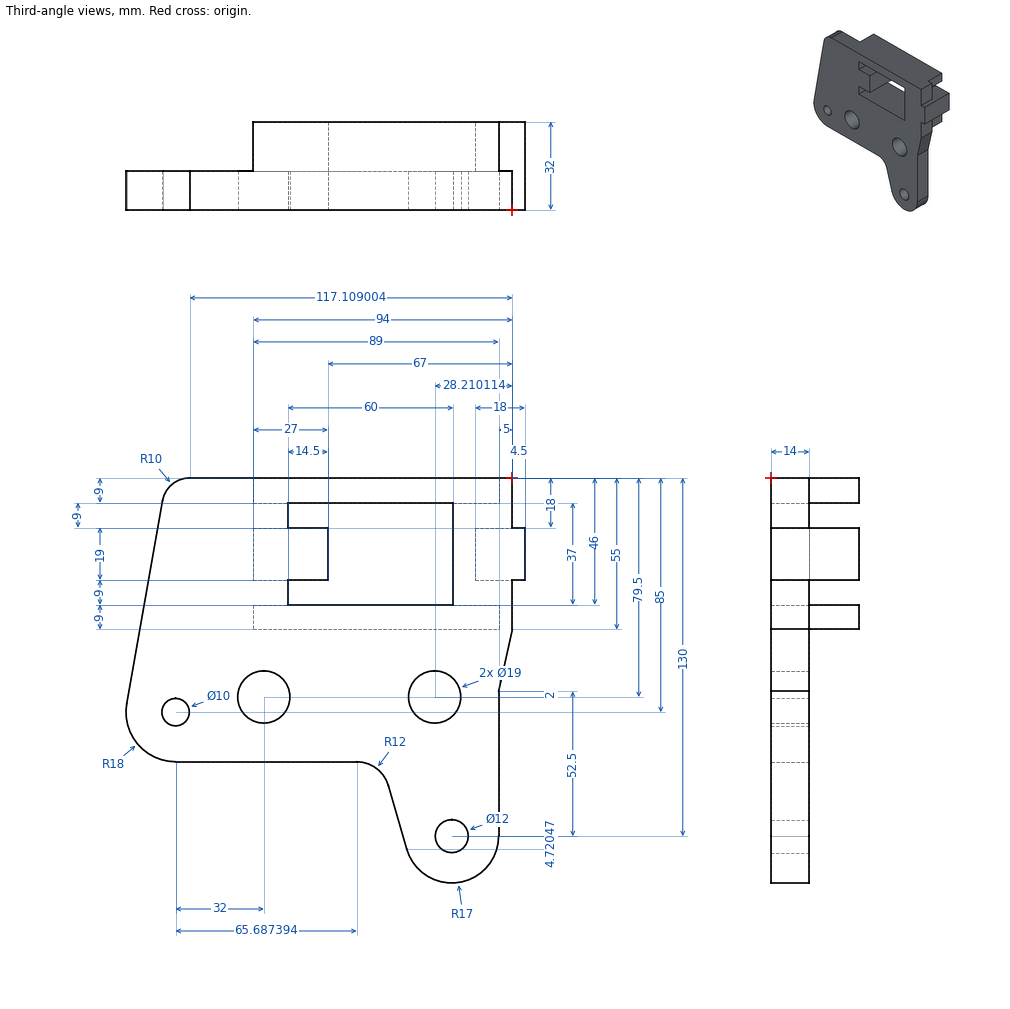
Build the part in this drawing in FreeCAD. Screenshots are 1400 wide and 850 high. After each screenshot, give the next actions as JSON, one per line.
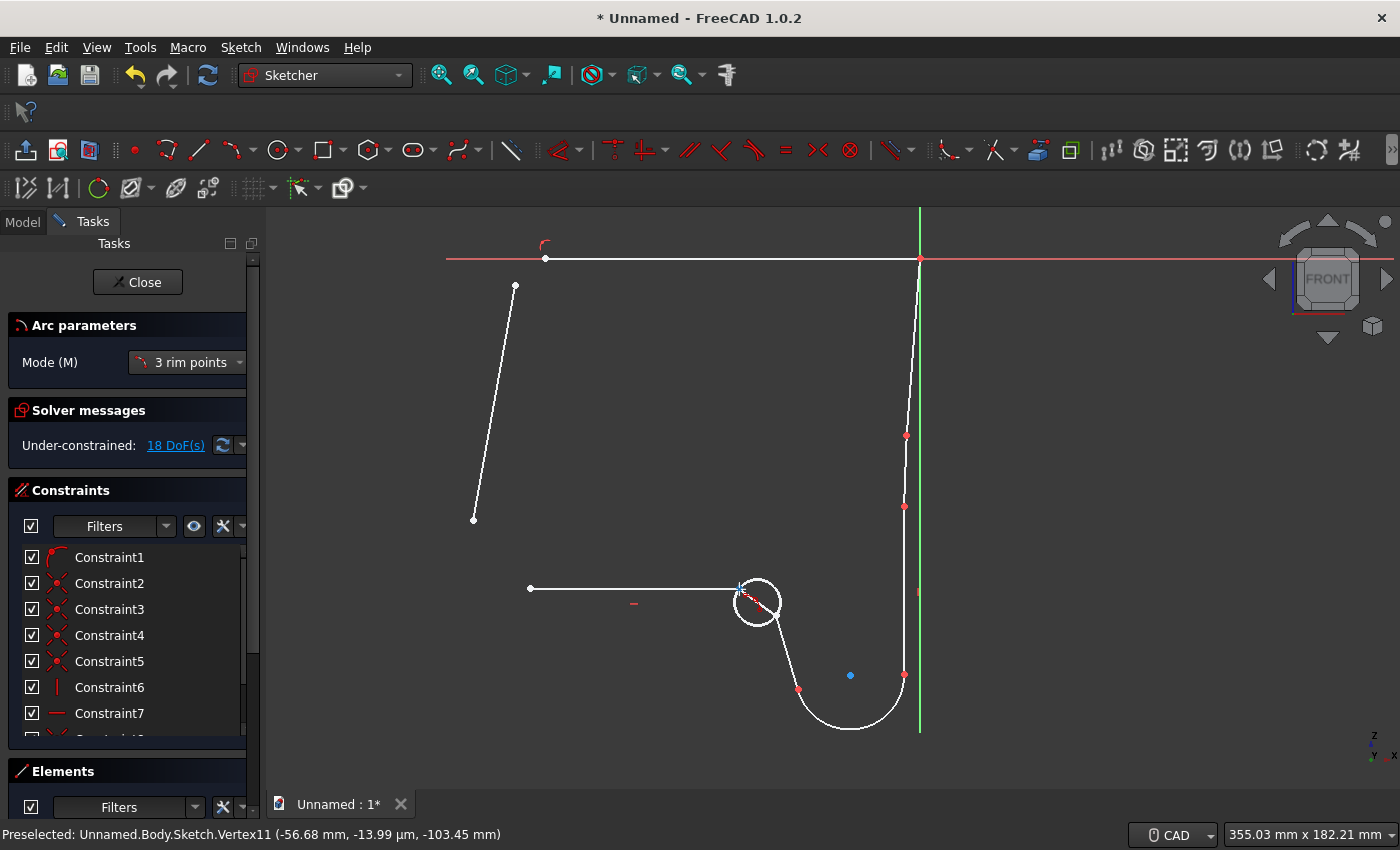
{"action": "scroll", "coordinate": [763, 595], "scroll_direction": "up", "scroll_amount": 4}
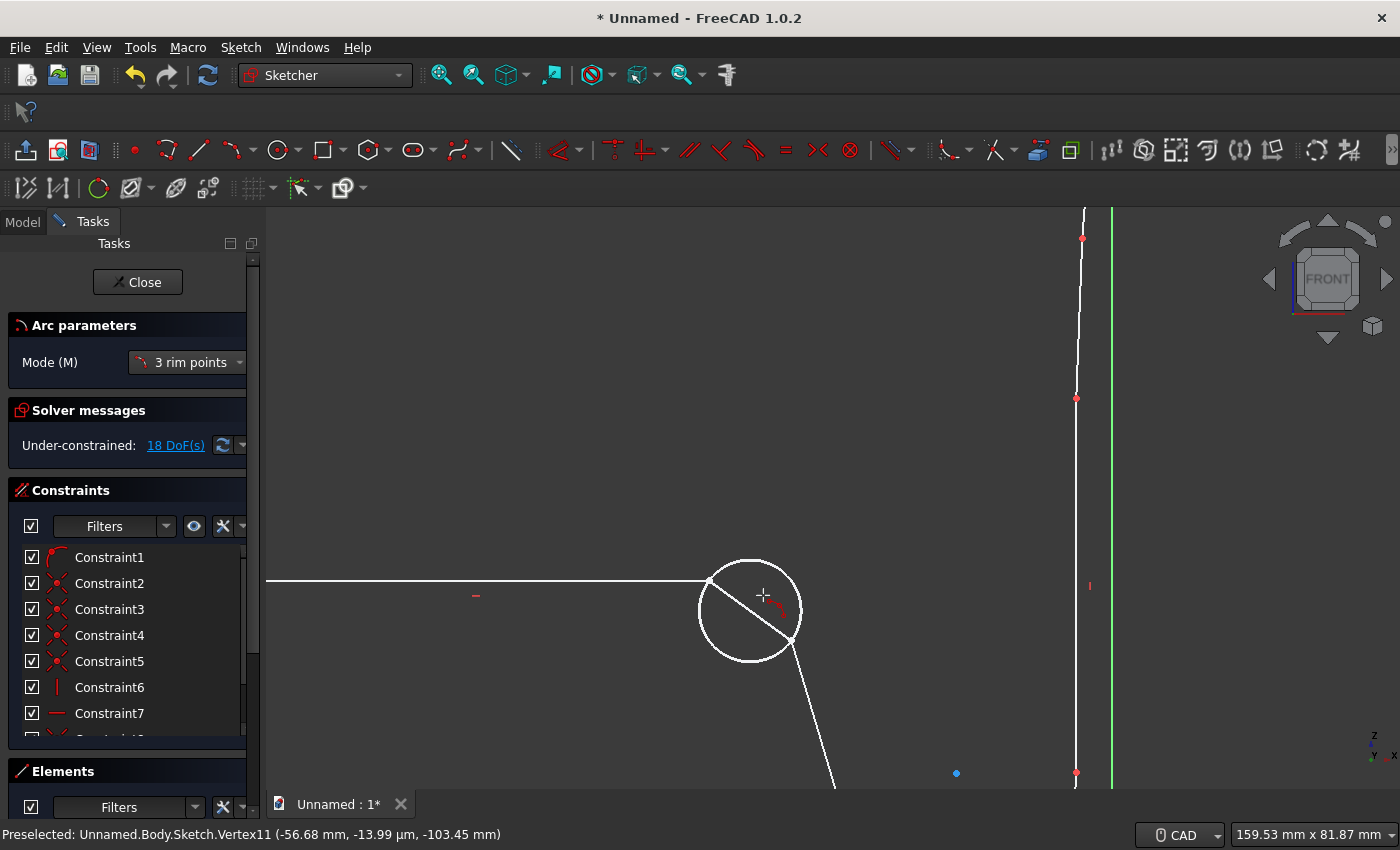
{"action": "left_click", "coordinate": [761, 595]}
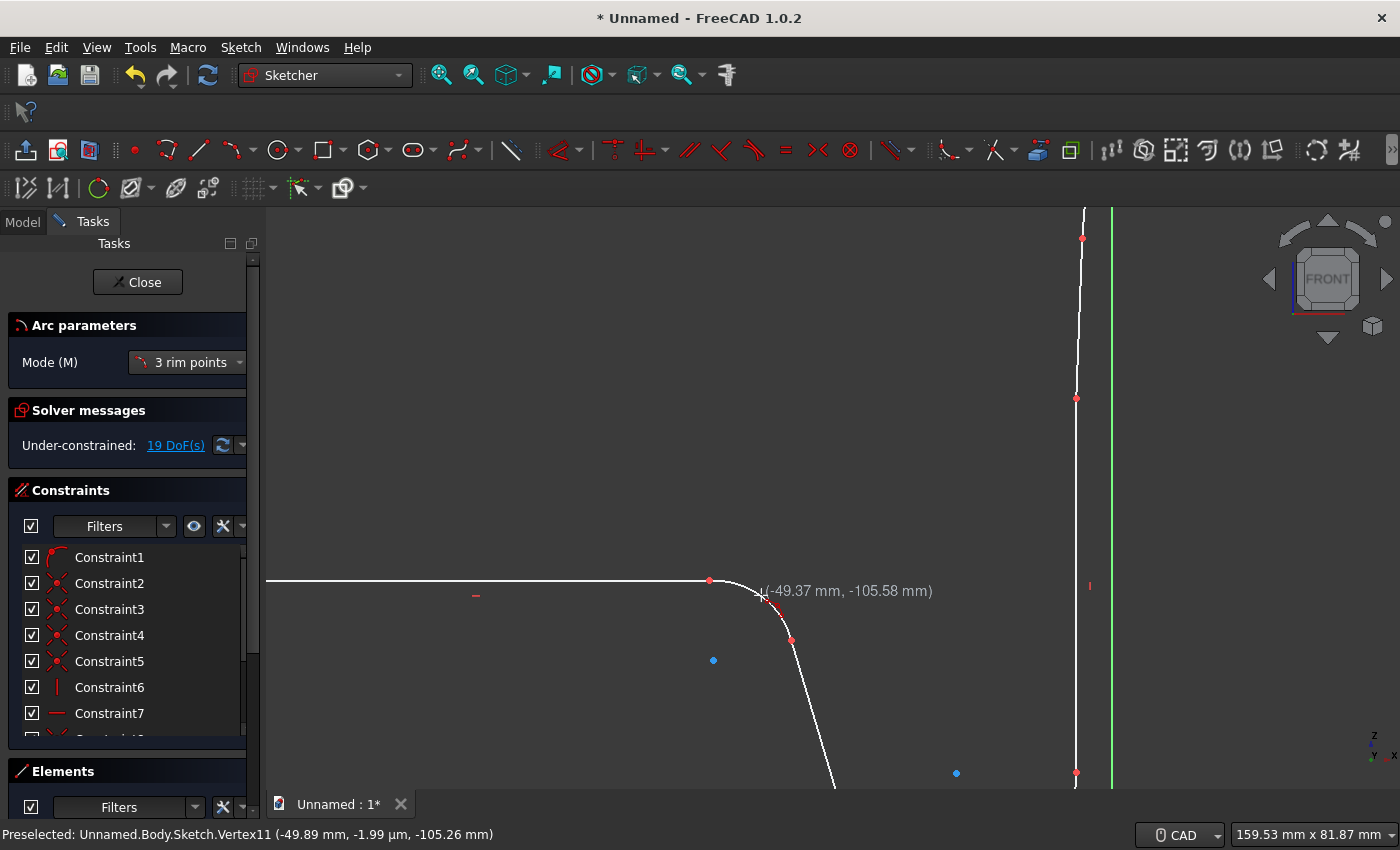
{"action": "scroll", "coordinate": [852, 574], "scroll_direction": "down", "scroll_amount": 5}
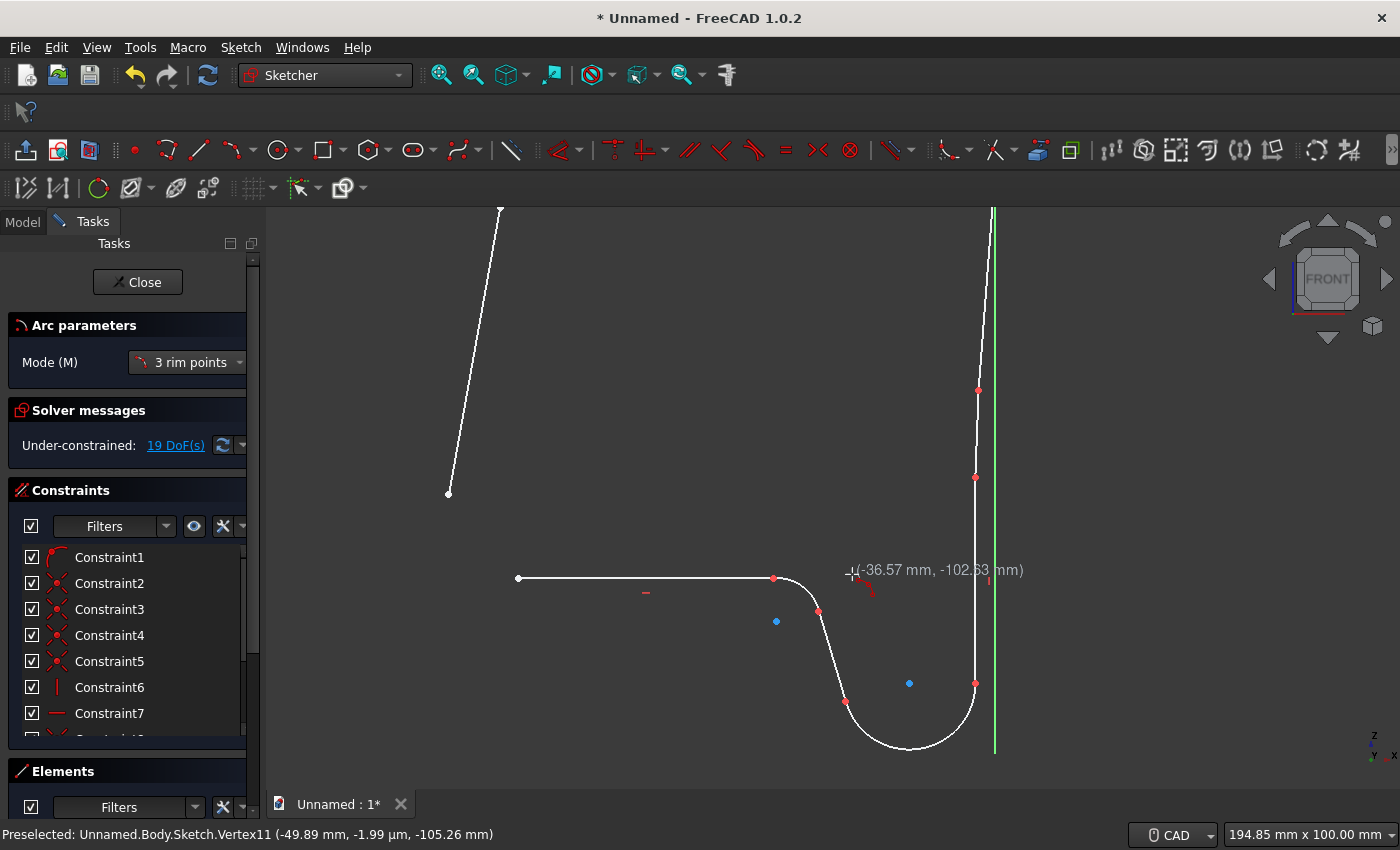
{"action": "left_click", "coordinate": [629, 577]}
{"action": "left_click", "coordinate": [582, 521]}
{"action": "left_click", "coordinate": [592, 559]}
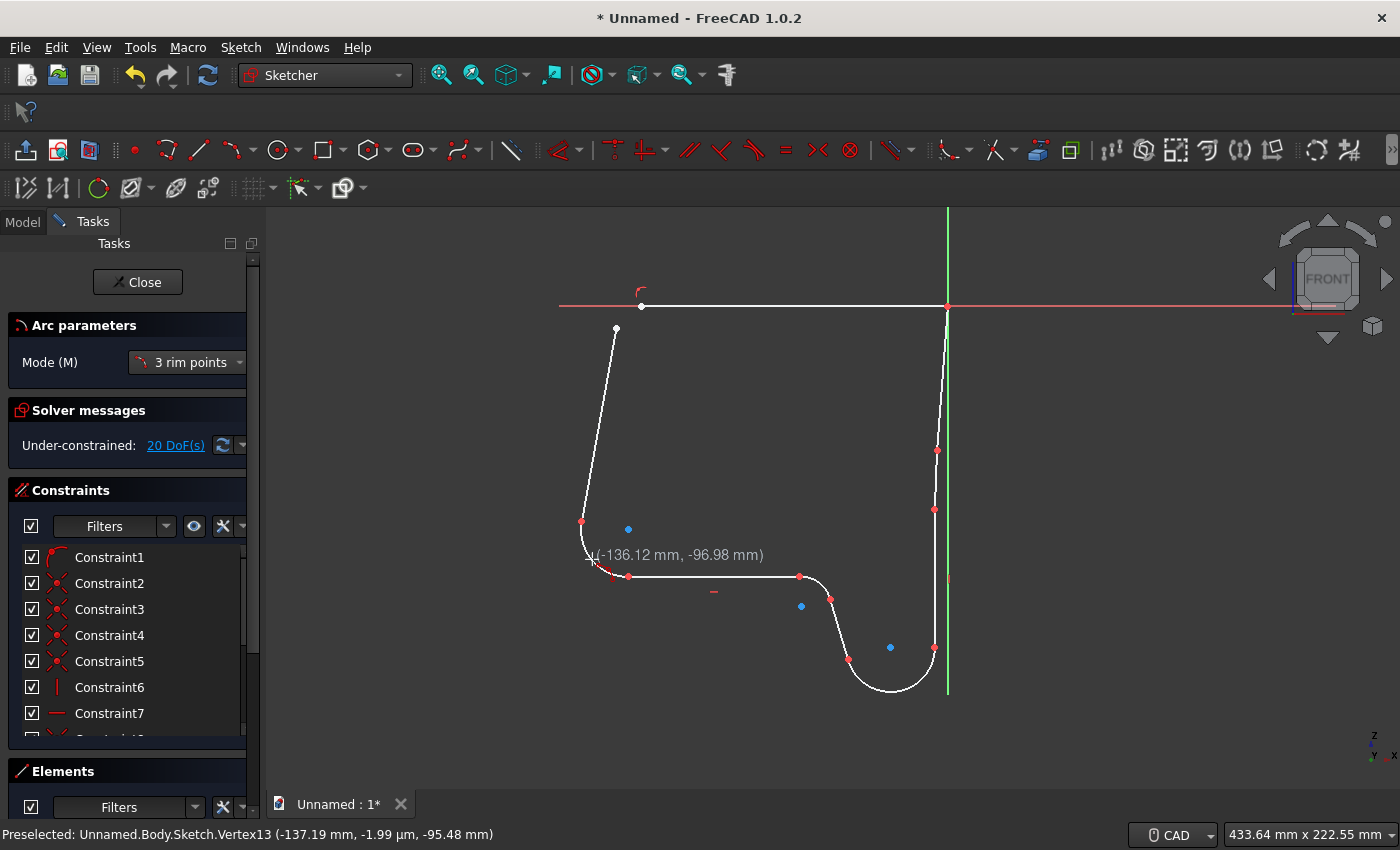
{"action": "left_click", "coordinate": [616, 329]}
{"action": "left_click", "coordinate": [641, 306]}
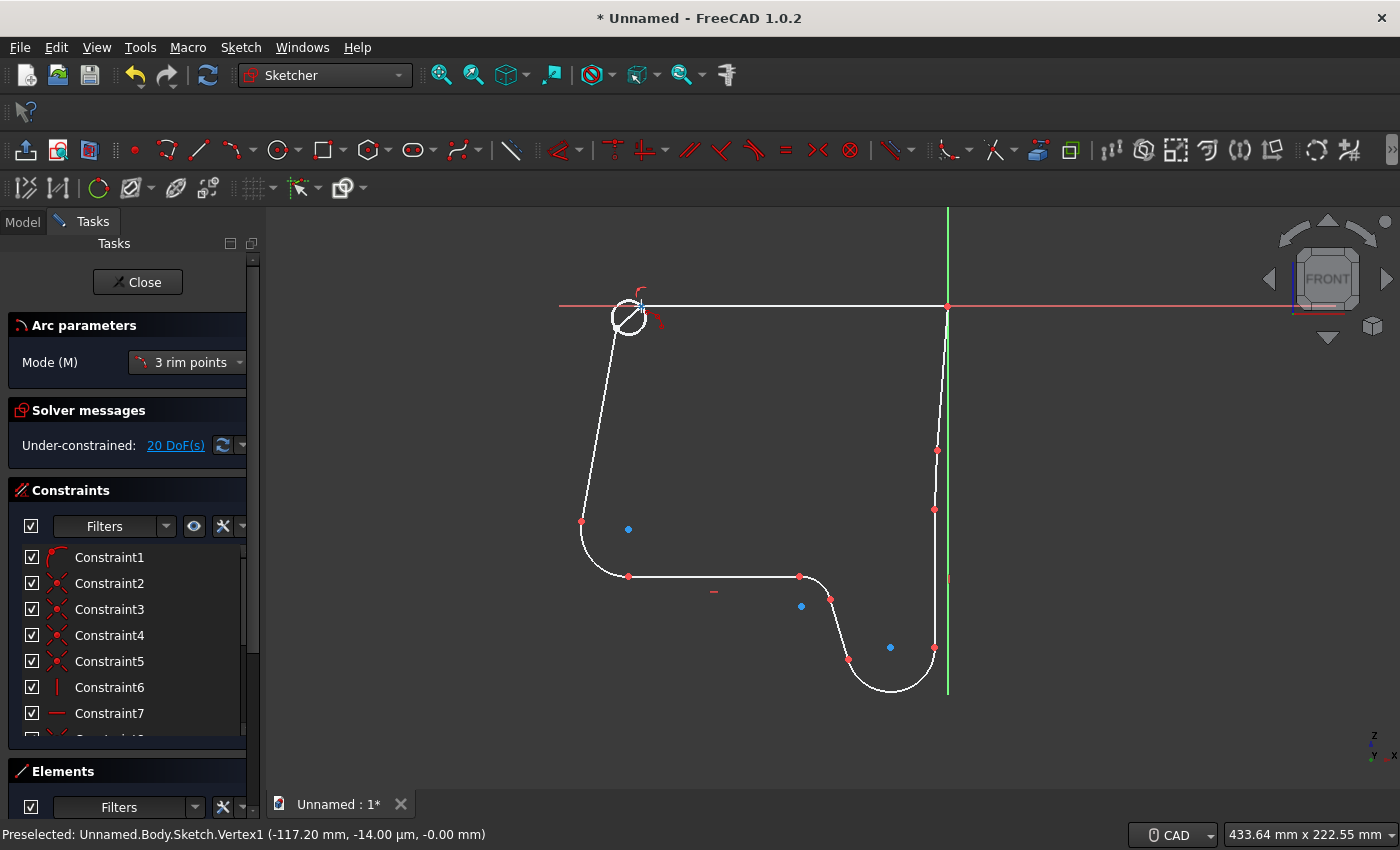
{"action": "scroll", "coordinate": [625, 313], "scroll_direction": "up", "scroll_amount": 5}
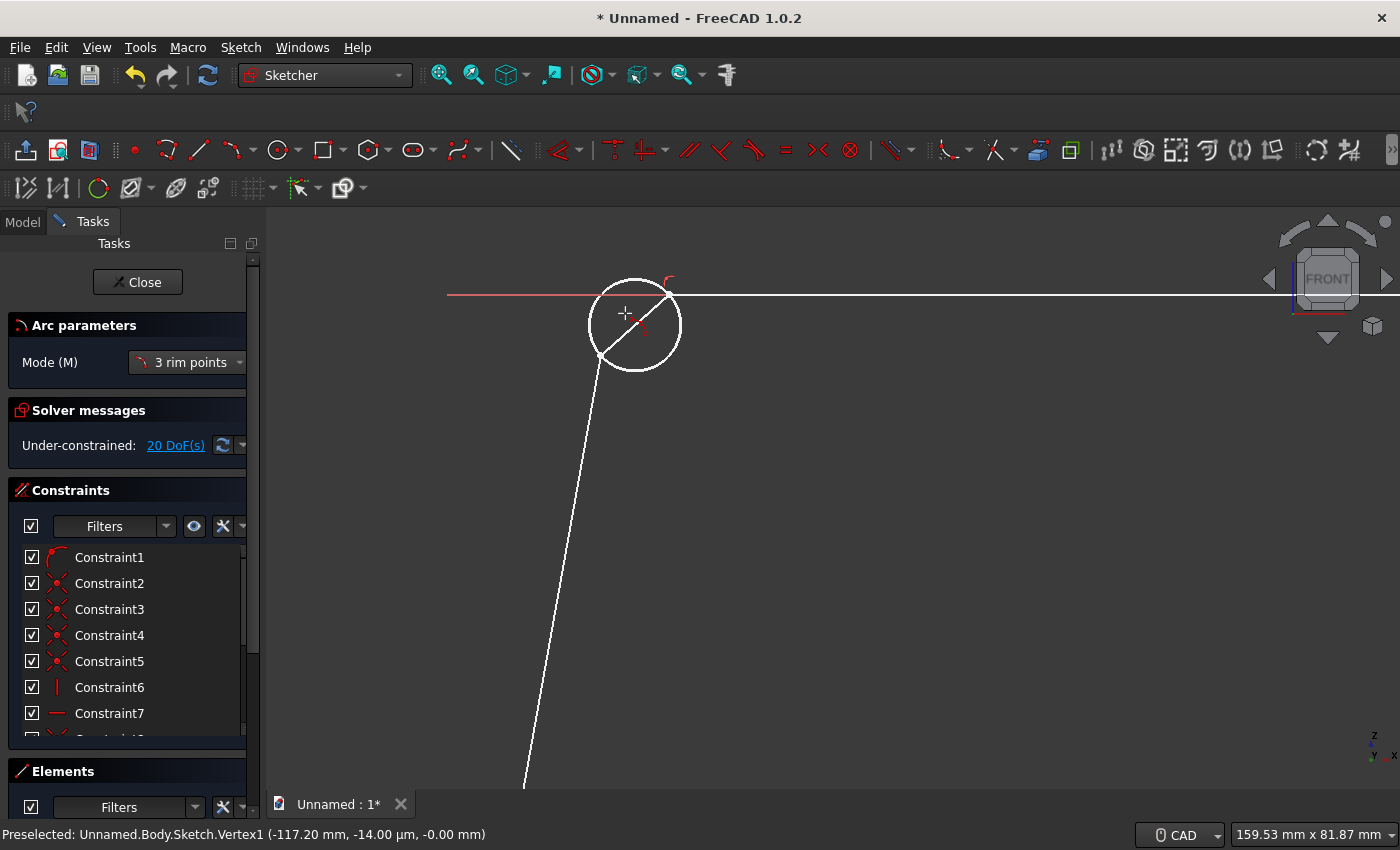
{"action": "left_click", "coordinate": [624, 311]}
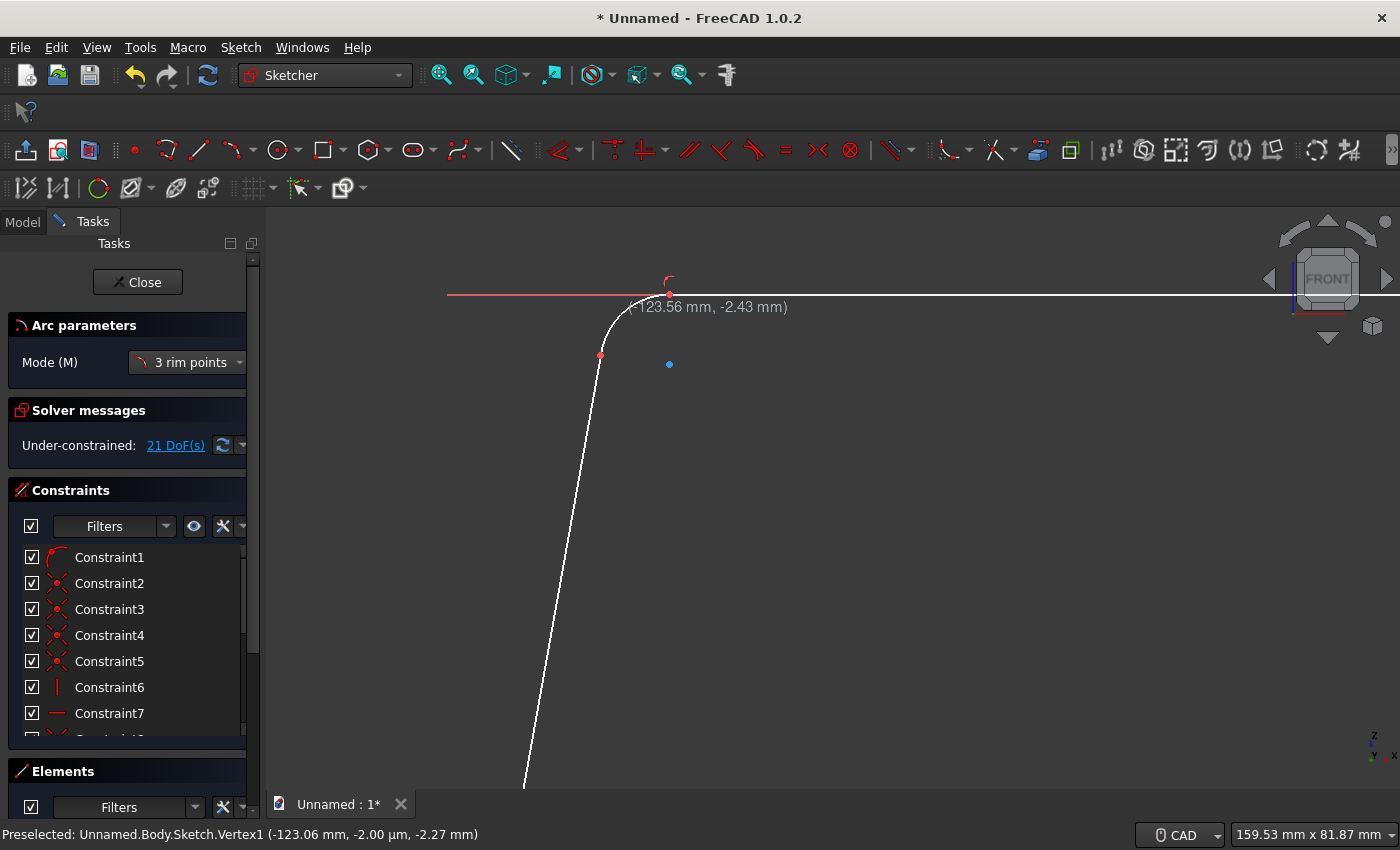
{"action": "key", "text": "g c"}